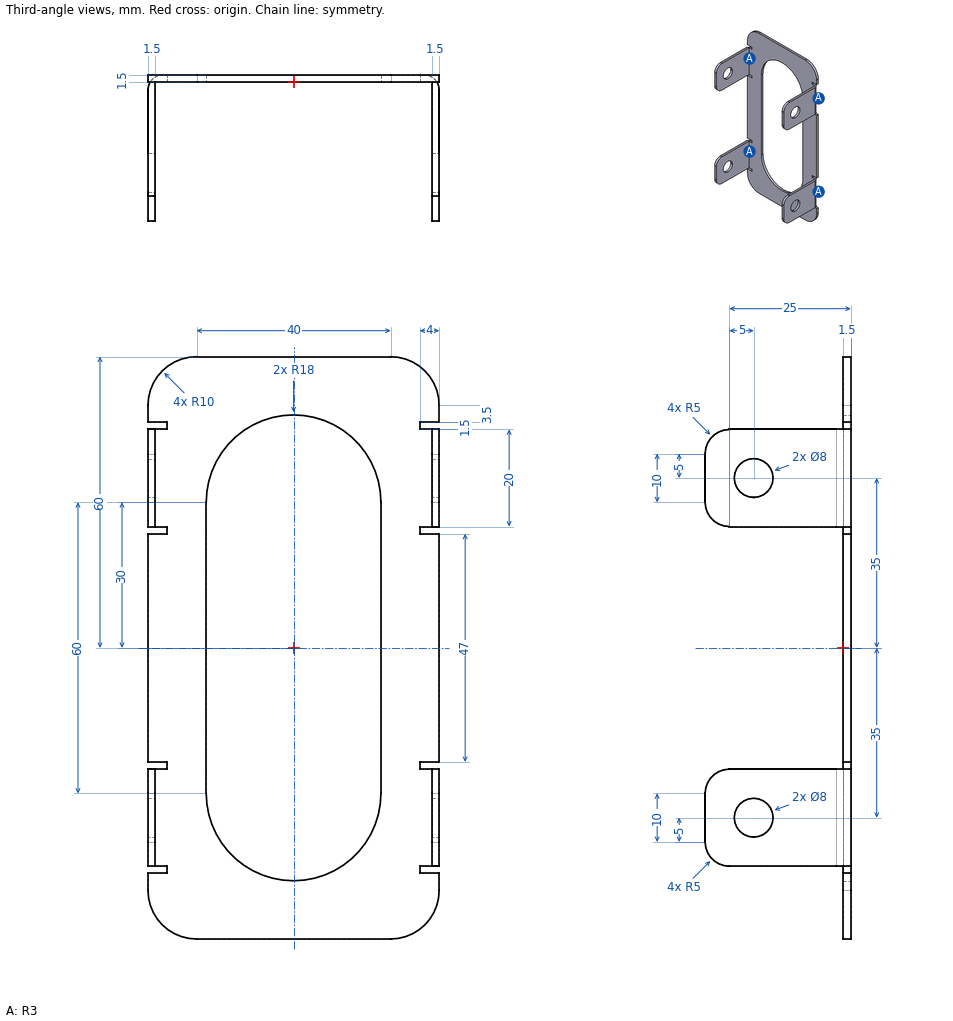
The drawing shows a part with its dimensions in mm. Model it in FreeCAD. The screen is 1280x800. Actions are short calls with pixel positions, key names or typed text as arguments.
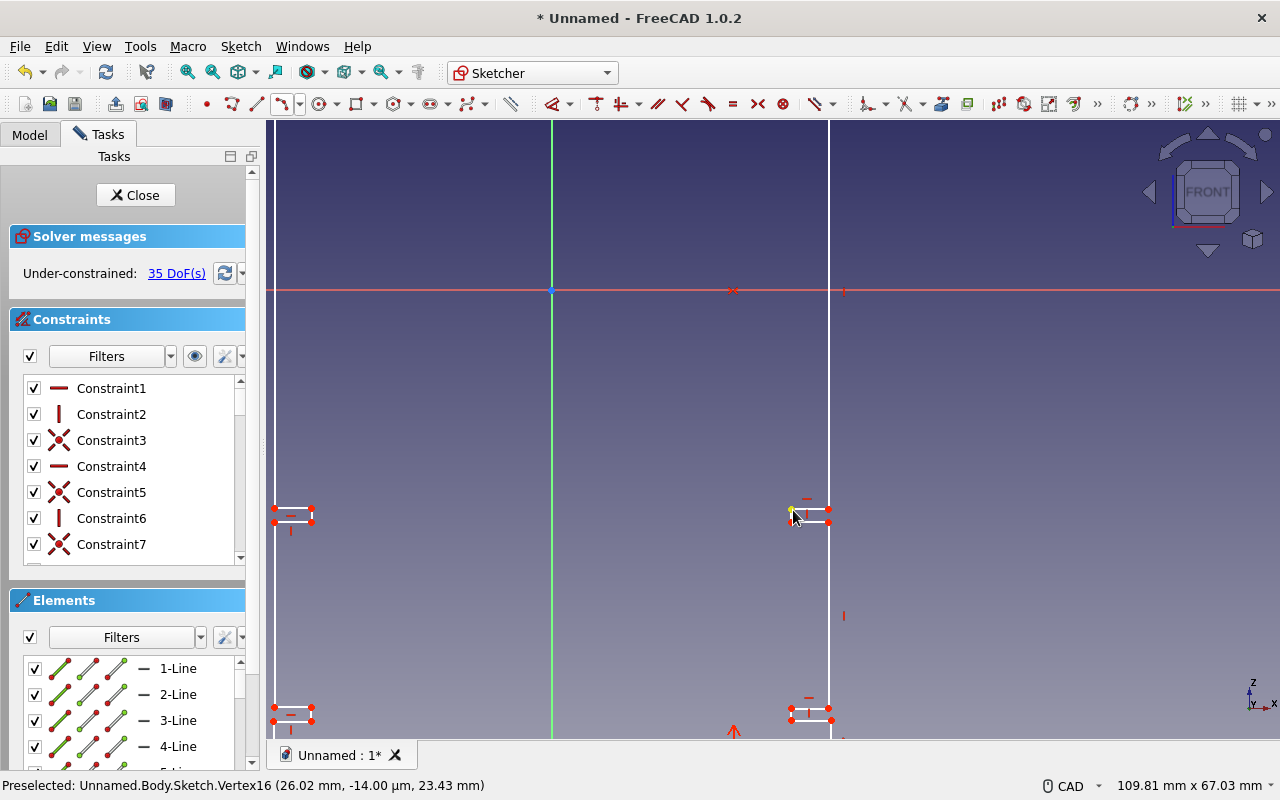
click(791, 509)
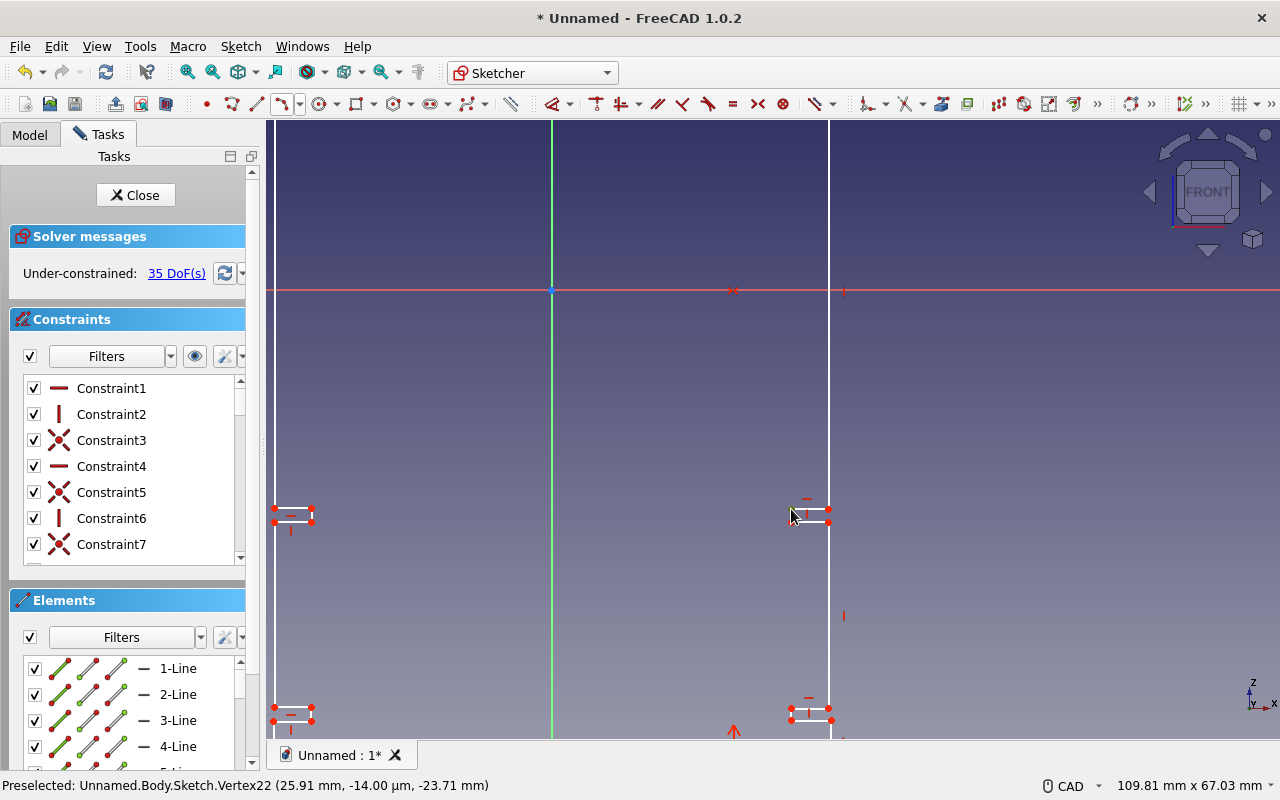
click(353, 290)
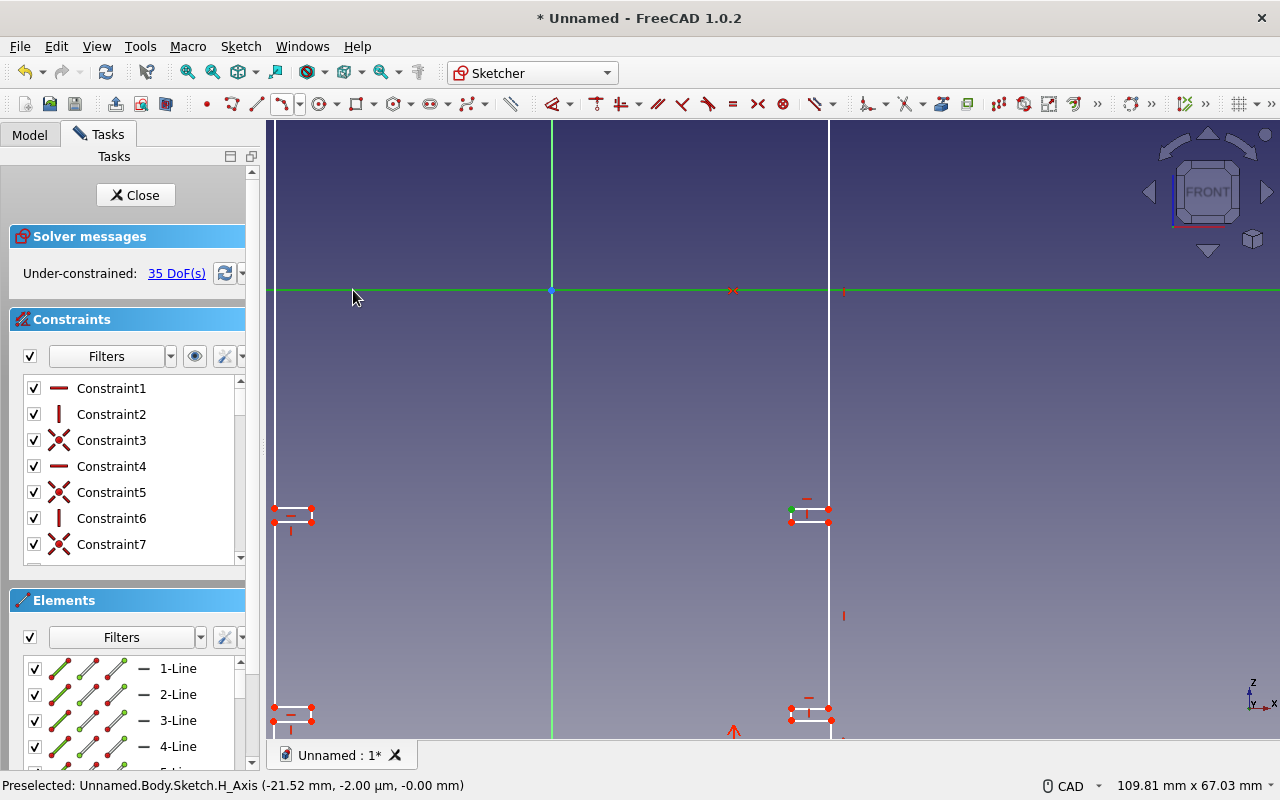
key(s)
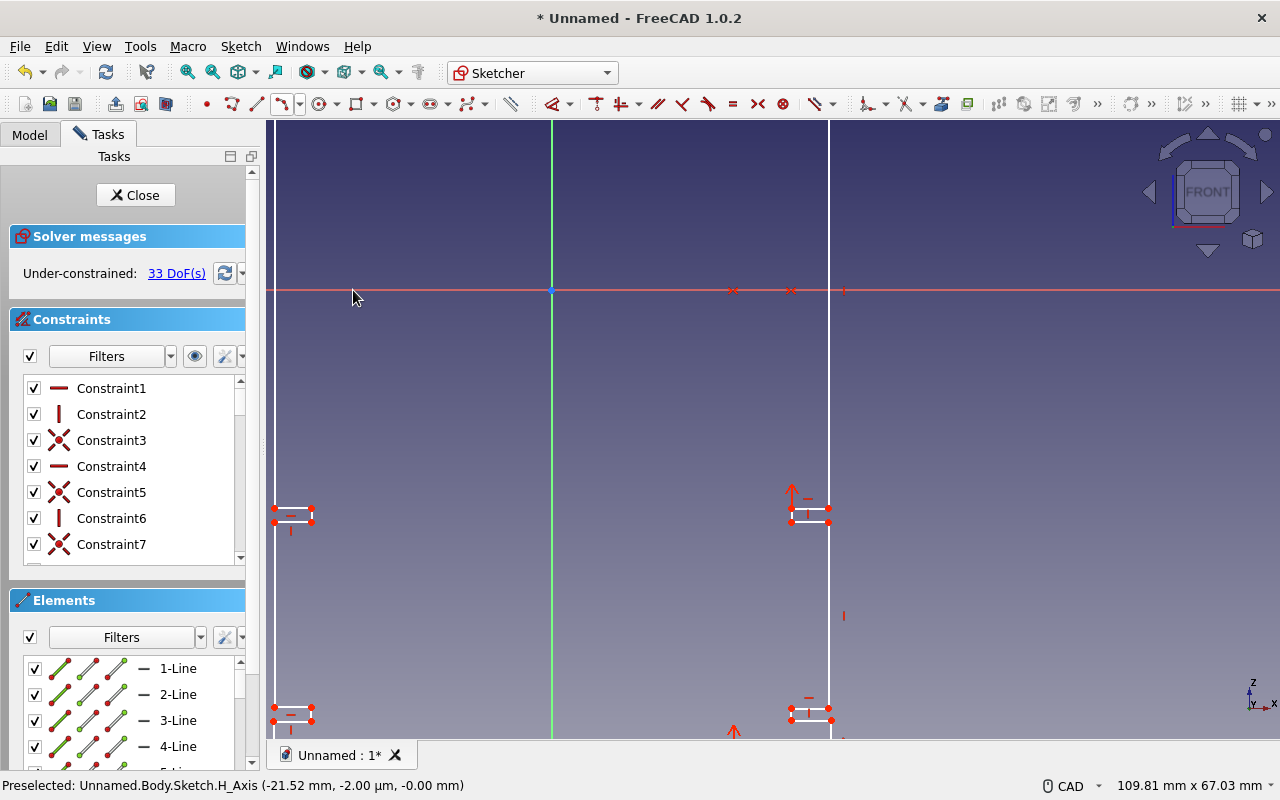
scroll(793, 510, down, 5)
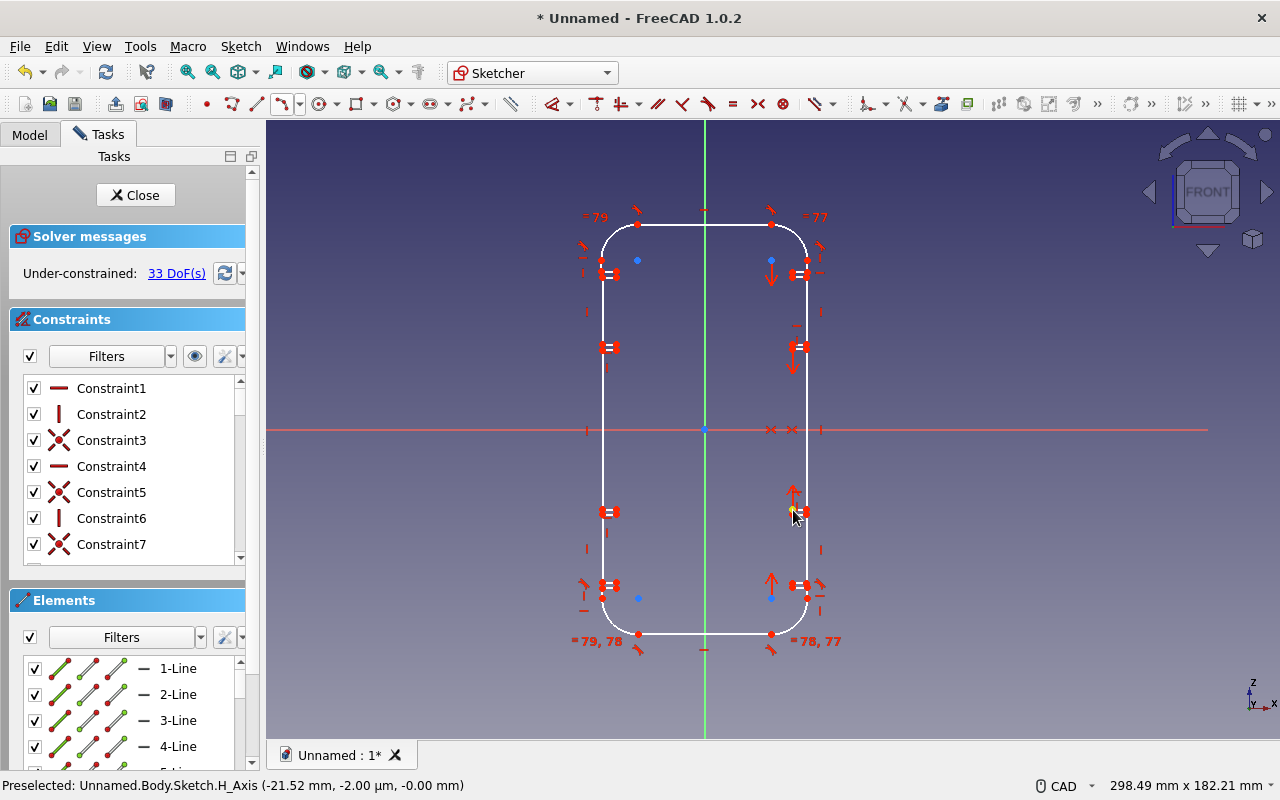
scroll(807, 345, up, 6)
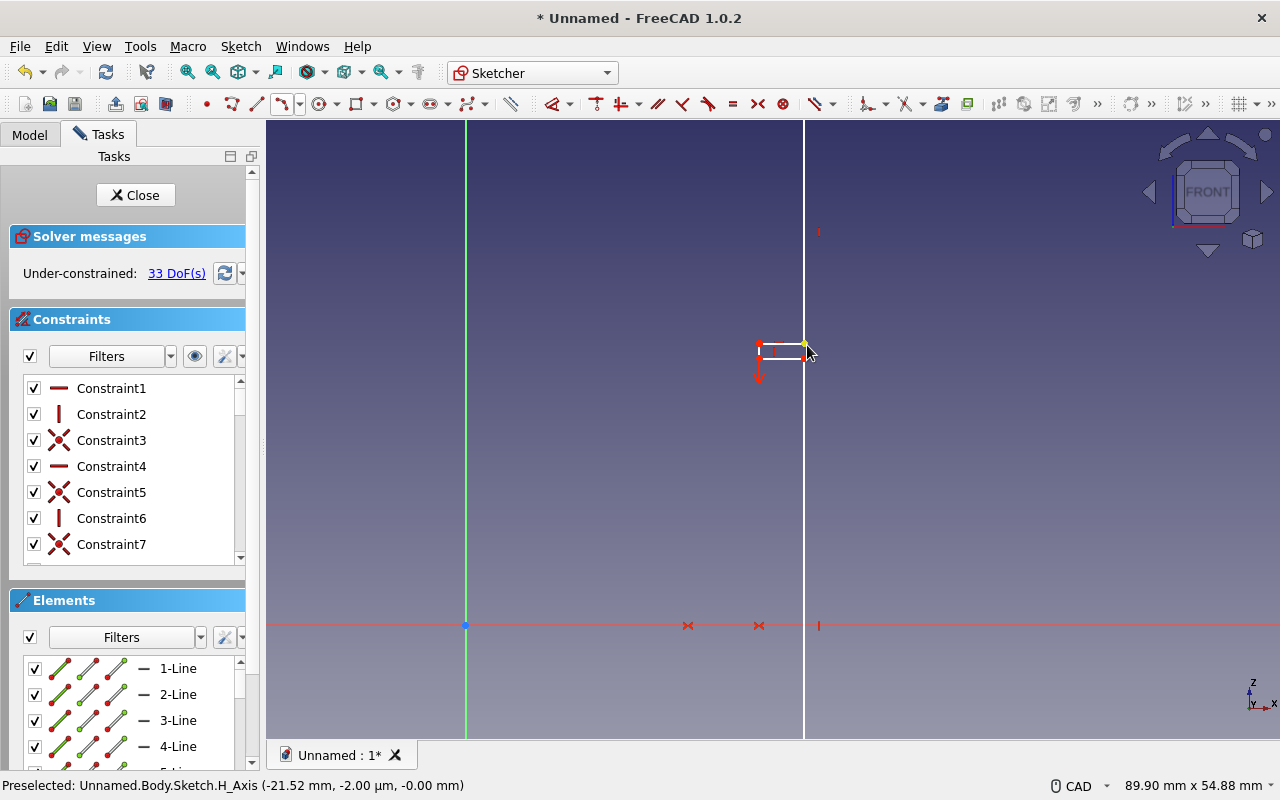
click(804, 344)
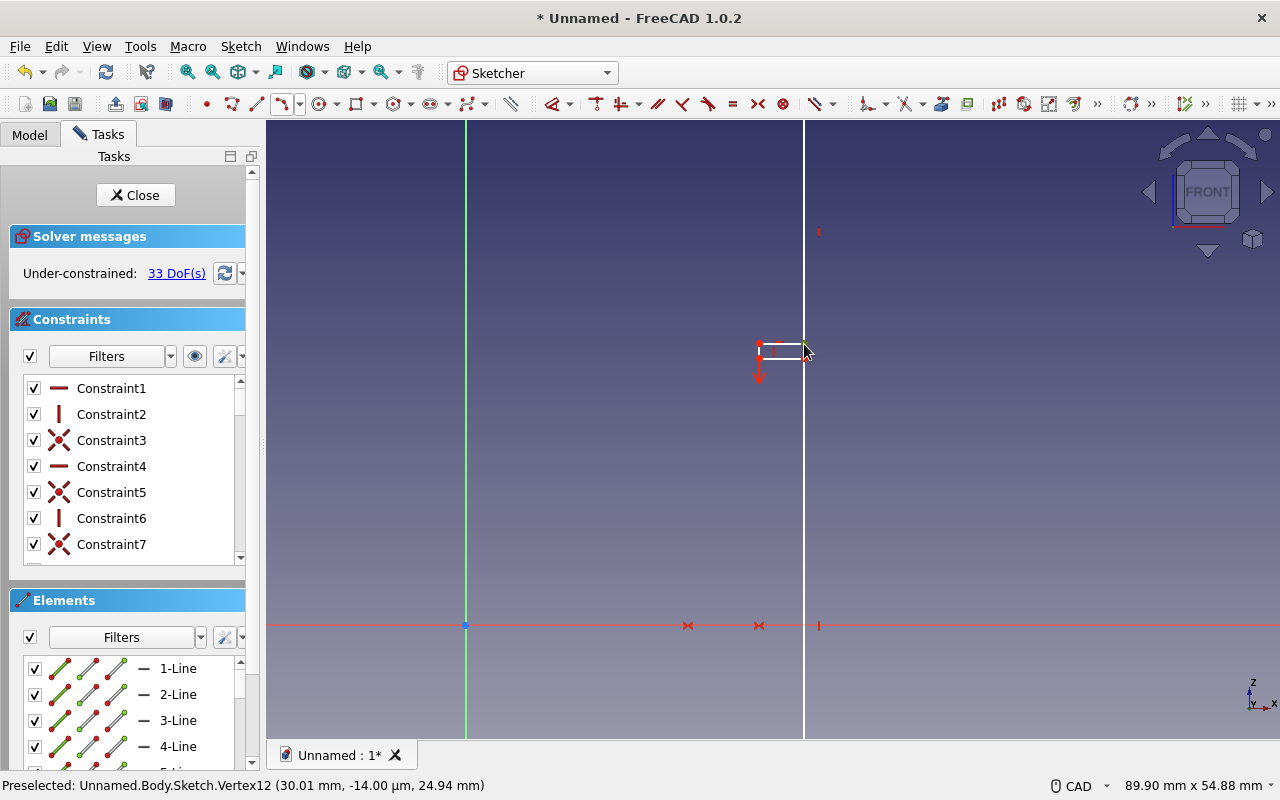
scroll(807, 345, down, 6)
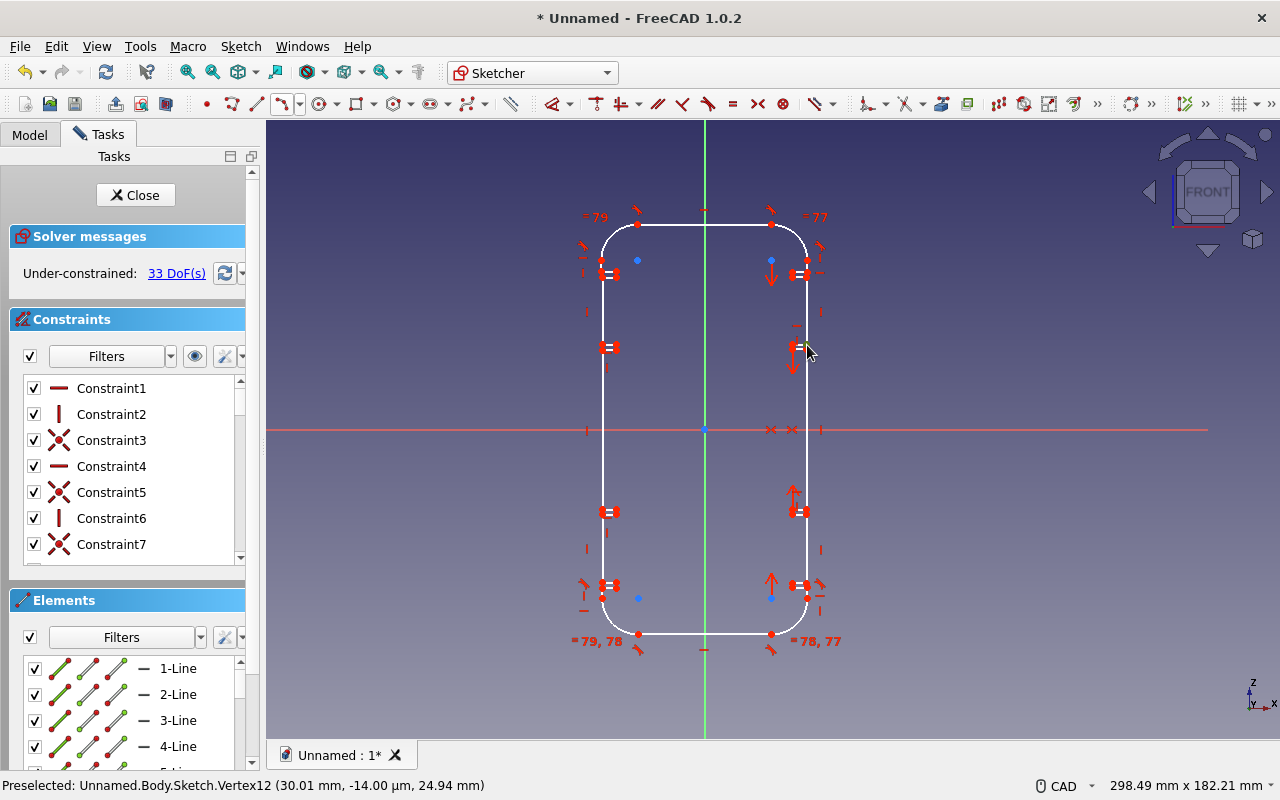
scroll(807, 515, up, 5)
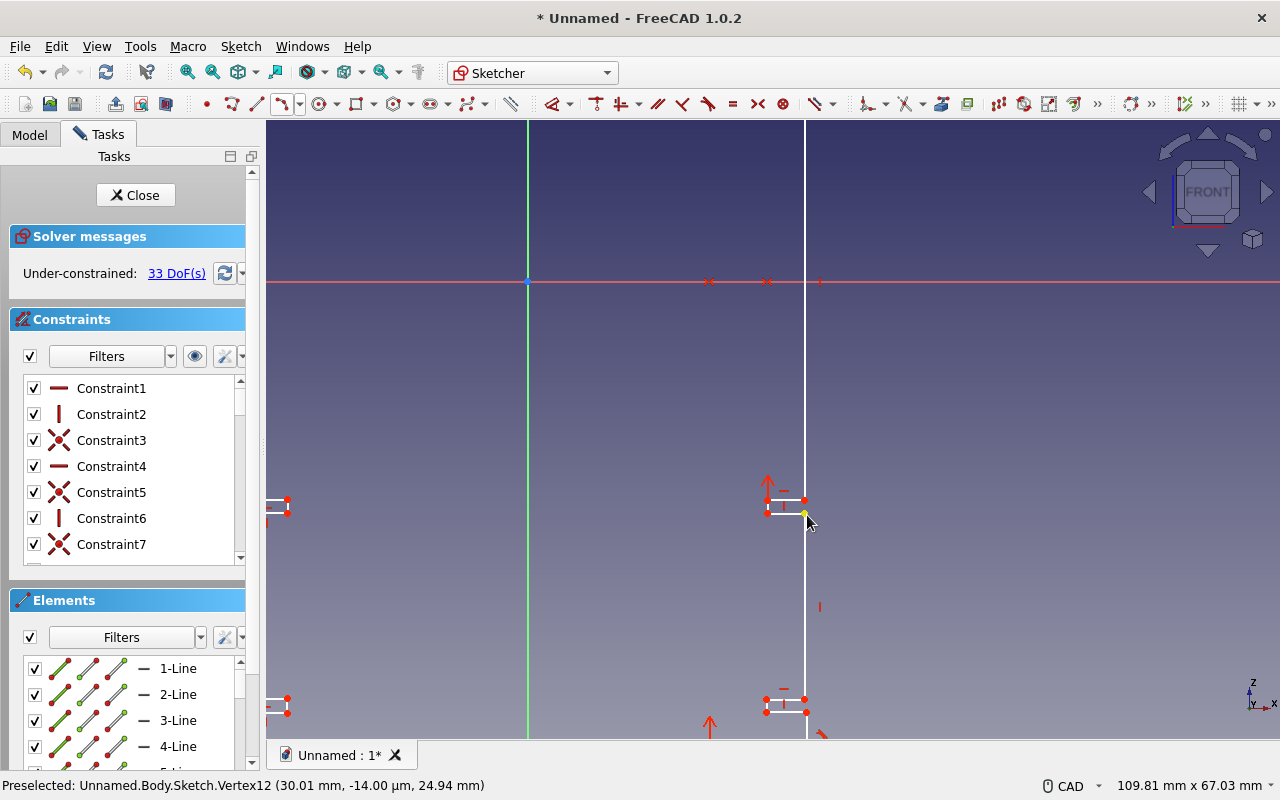
click(805, 514)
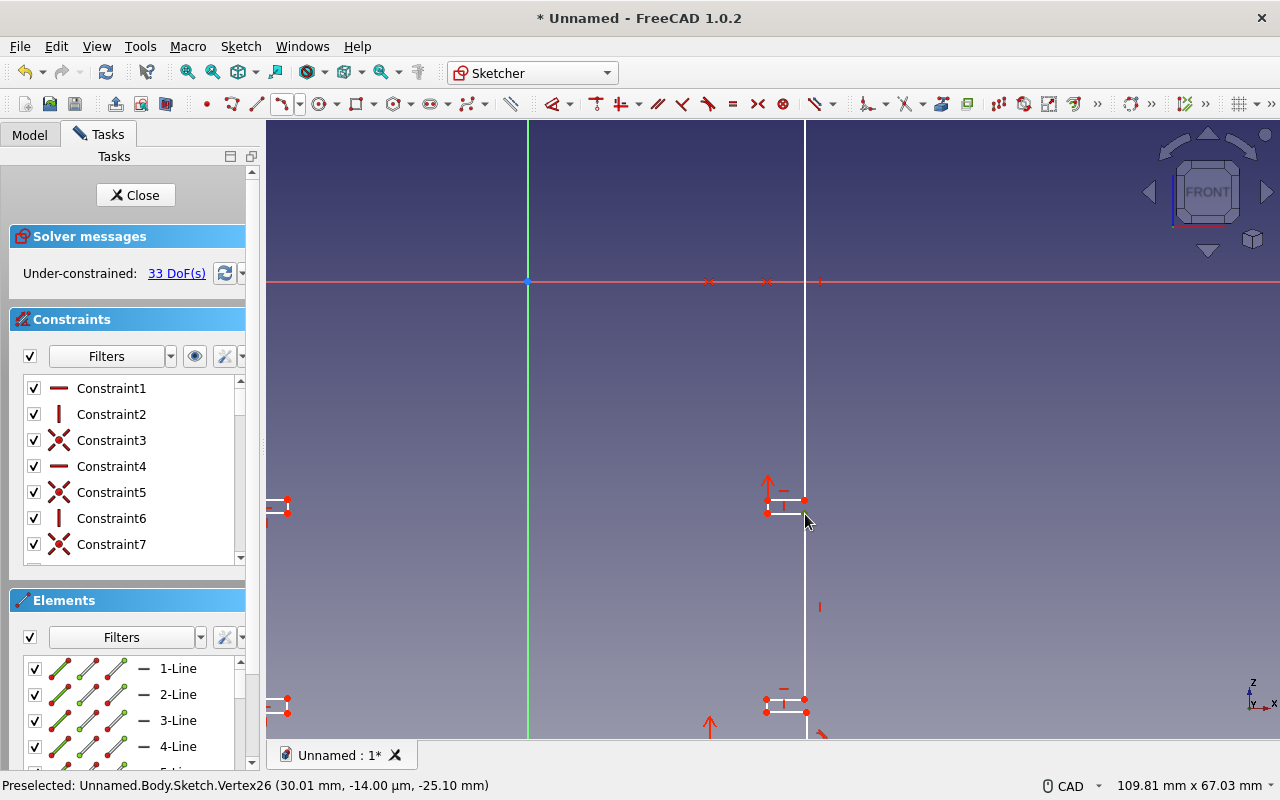
click(353, 282)